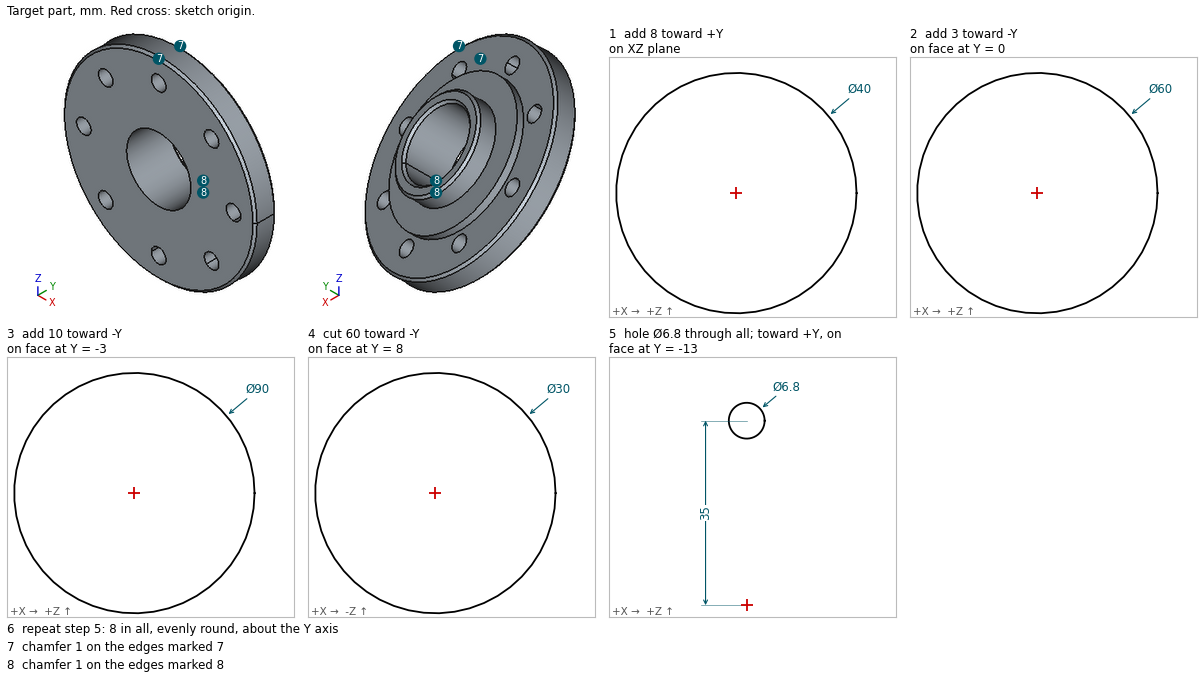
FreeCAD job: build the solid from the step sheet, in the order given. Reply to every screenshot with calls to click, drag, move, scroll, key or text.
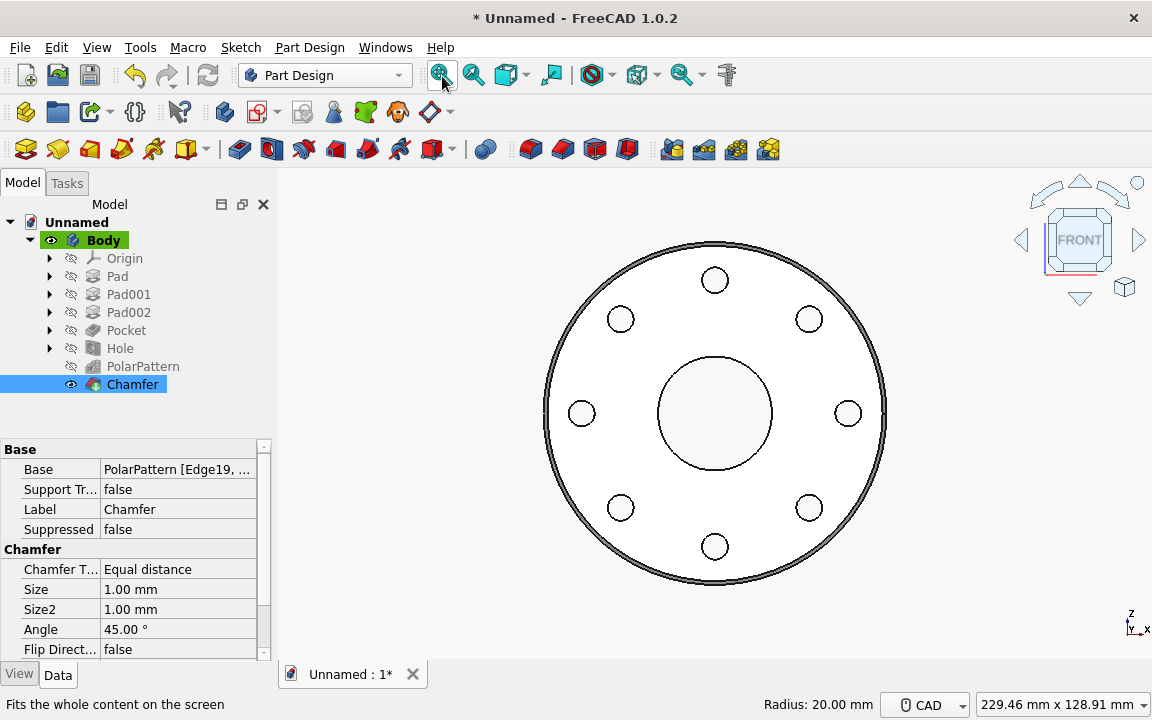
key(3)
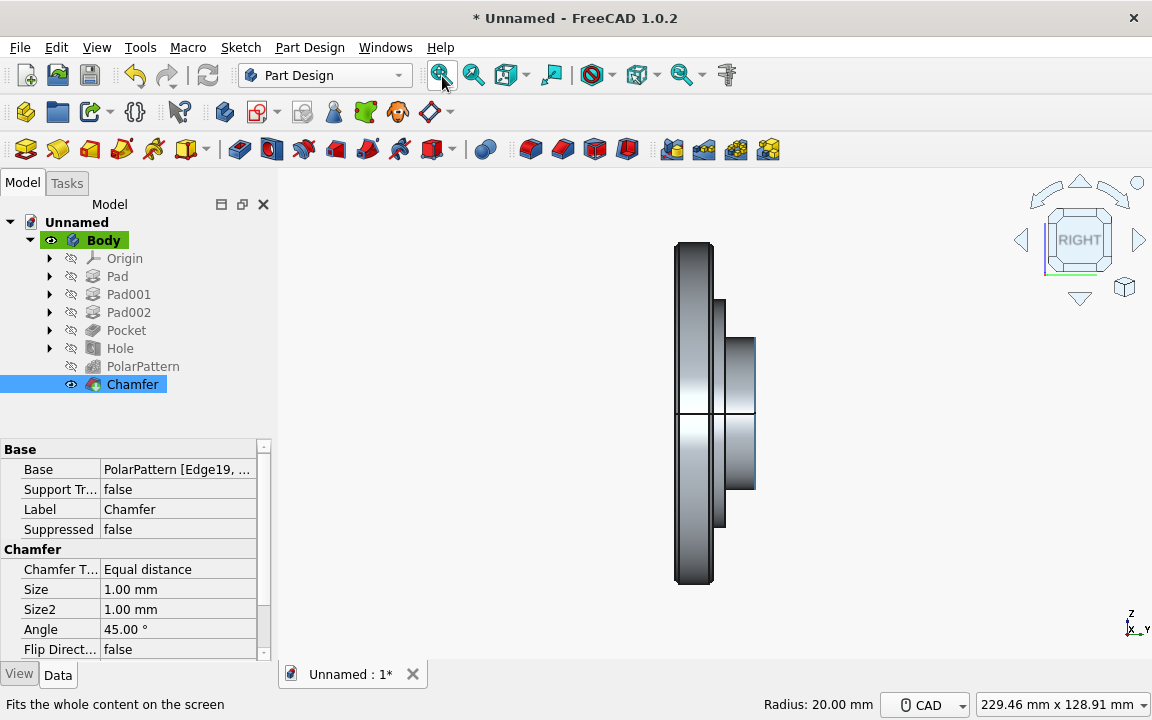
key(5)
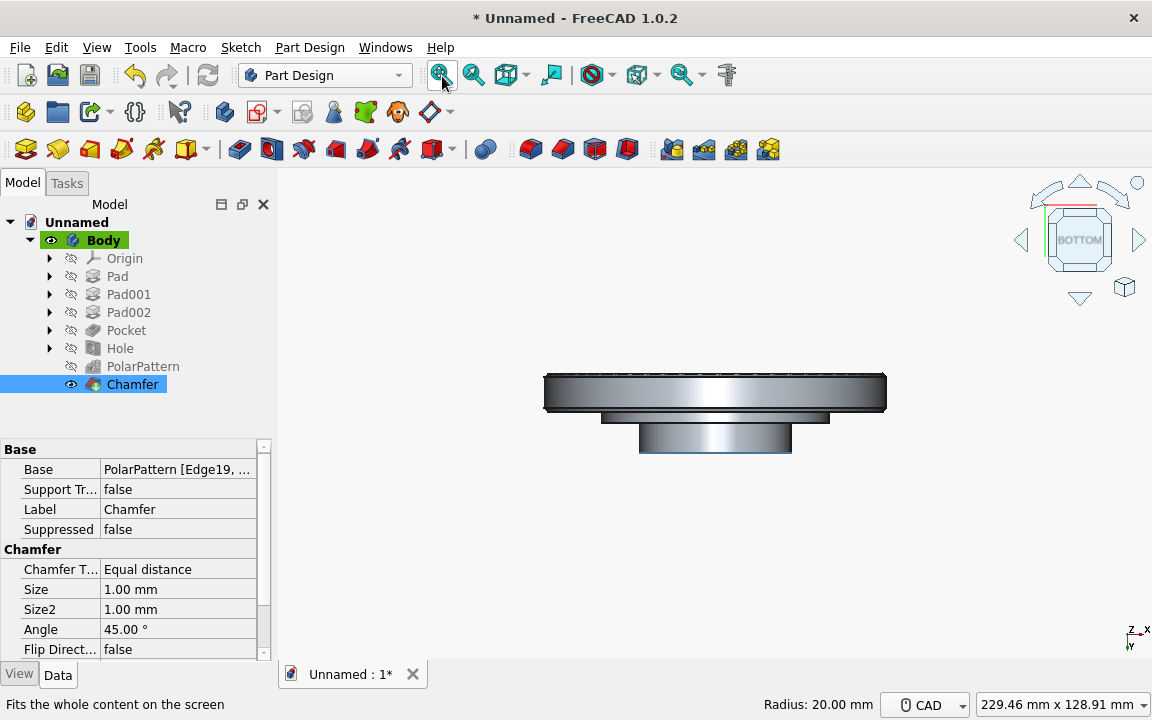
click(442, 76)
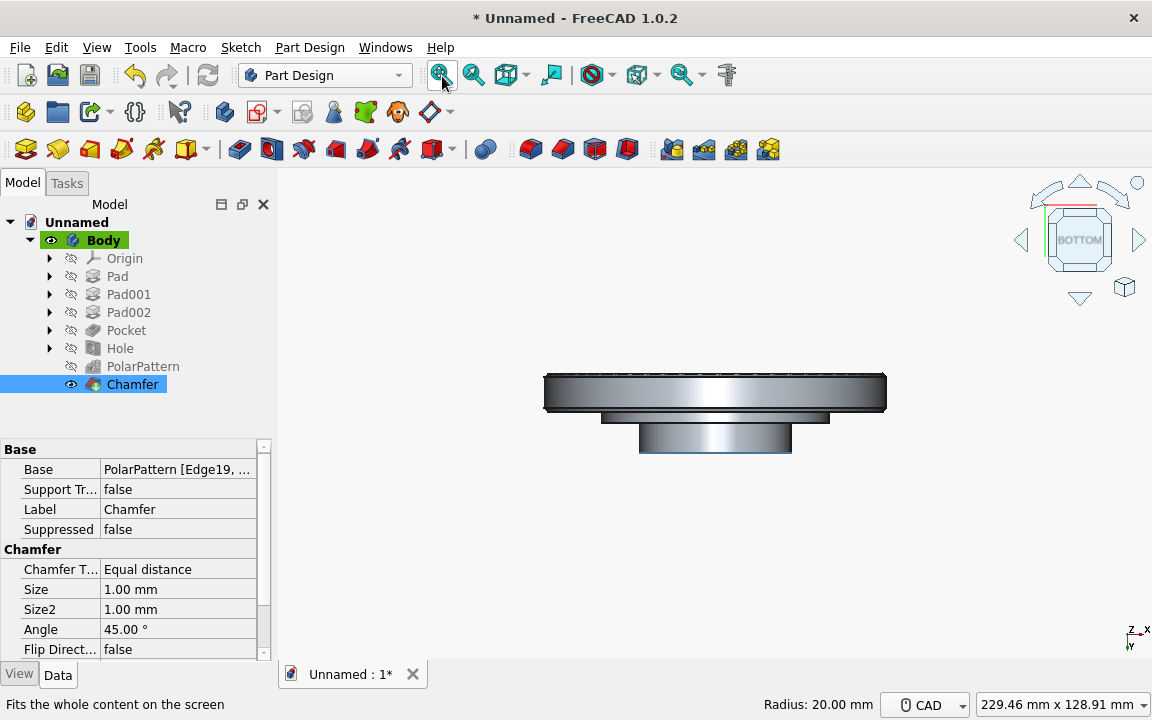
key(4)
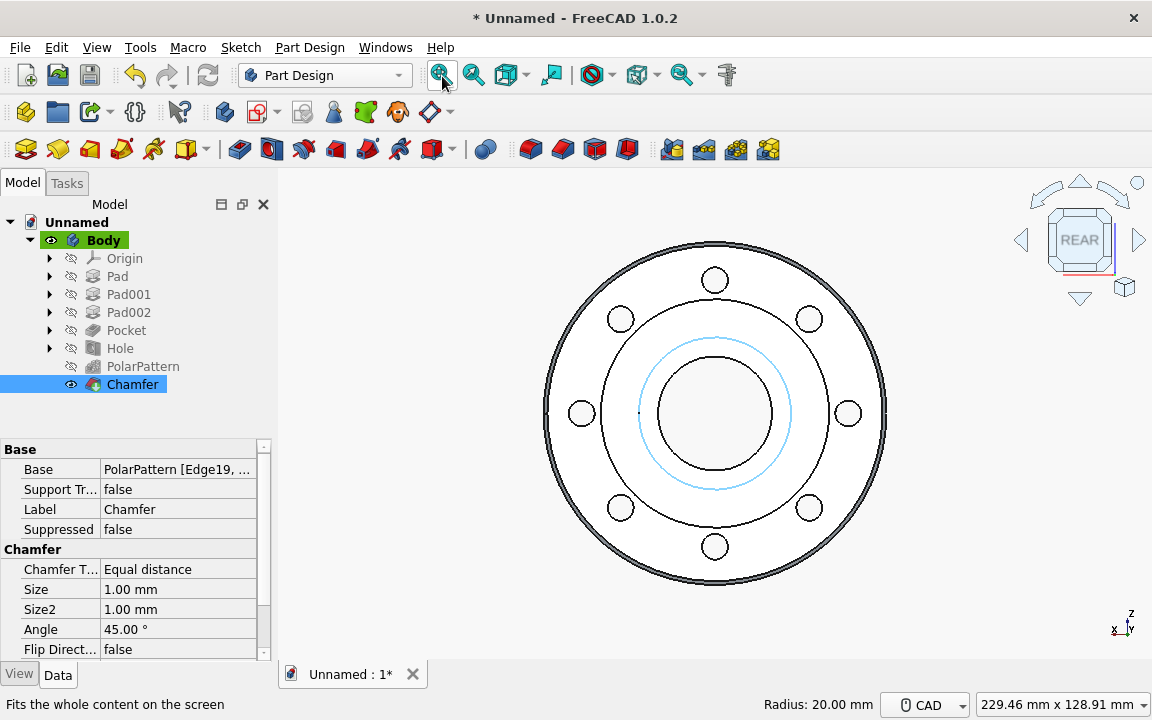
click(761, 379, ctrl)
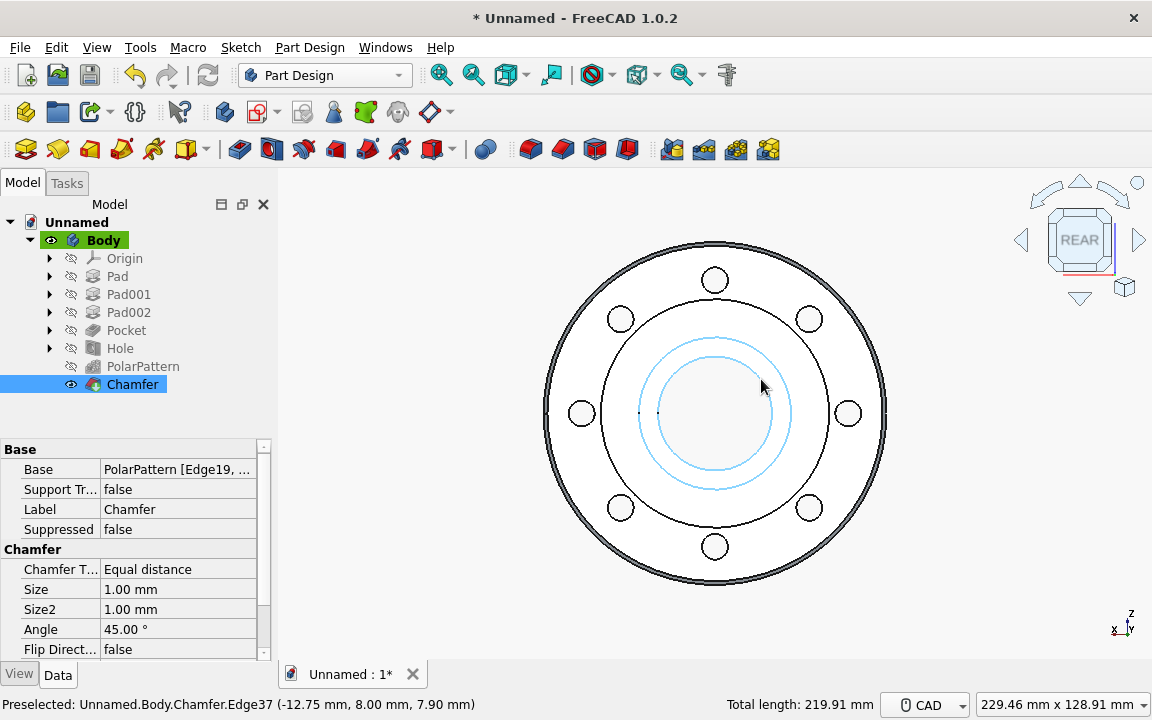
click(564, 150)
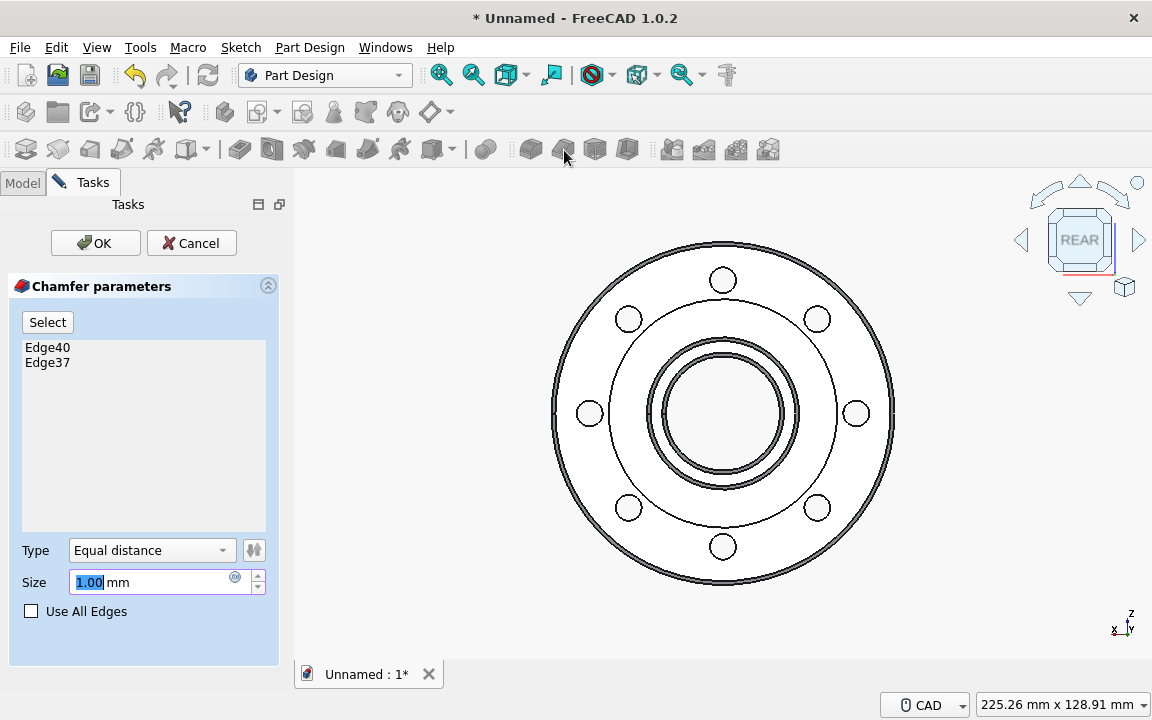
text(1)
key(Tab)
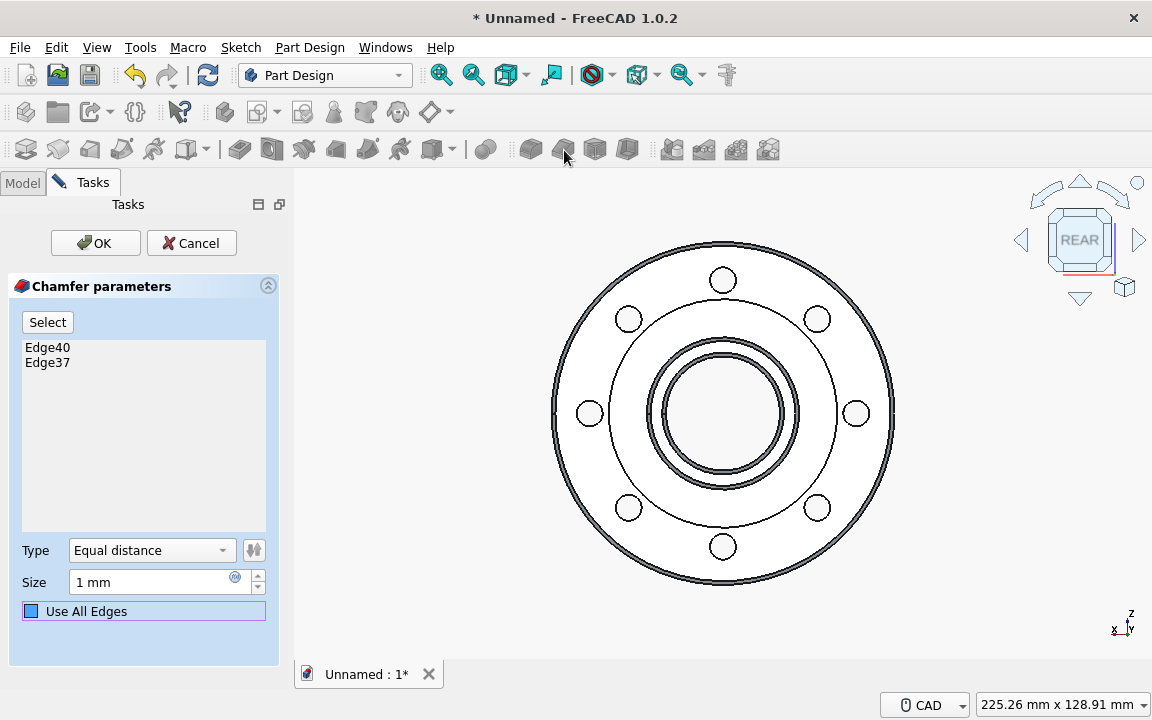
click(96, 243)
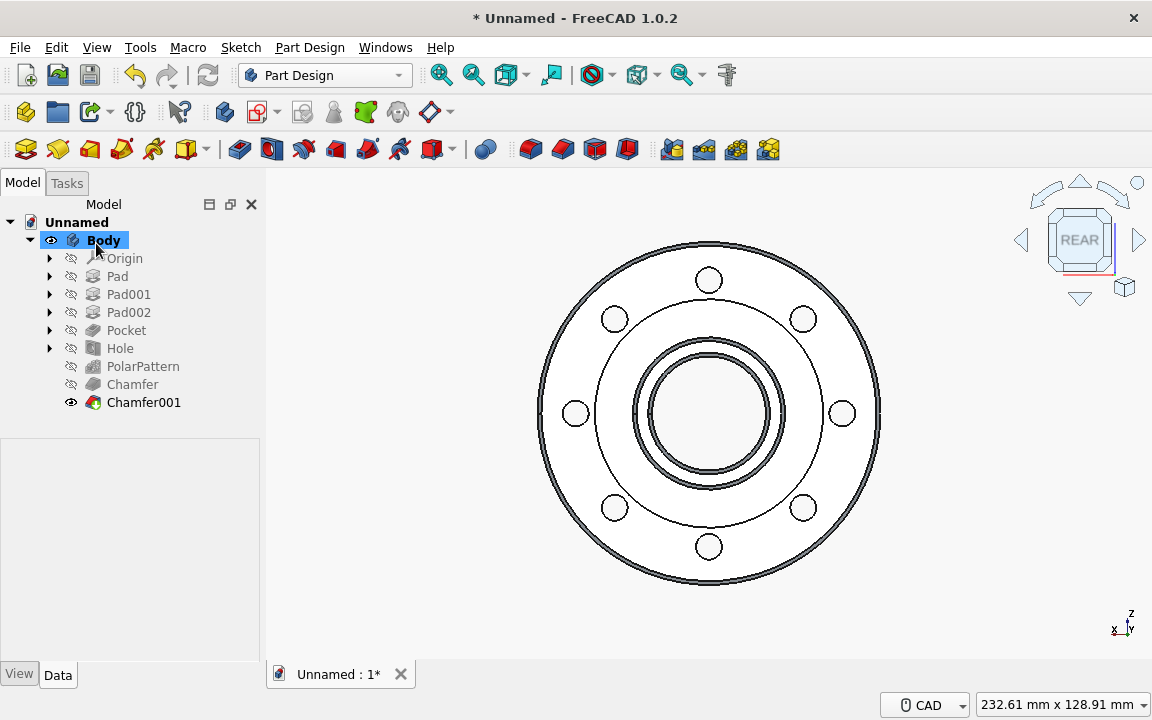
key(0)